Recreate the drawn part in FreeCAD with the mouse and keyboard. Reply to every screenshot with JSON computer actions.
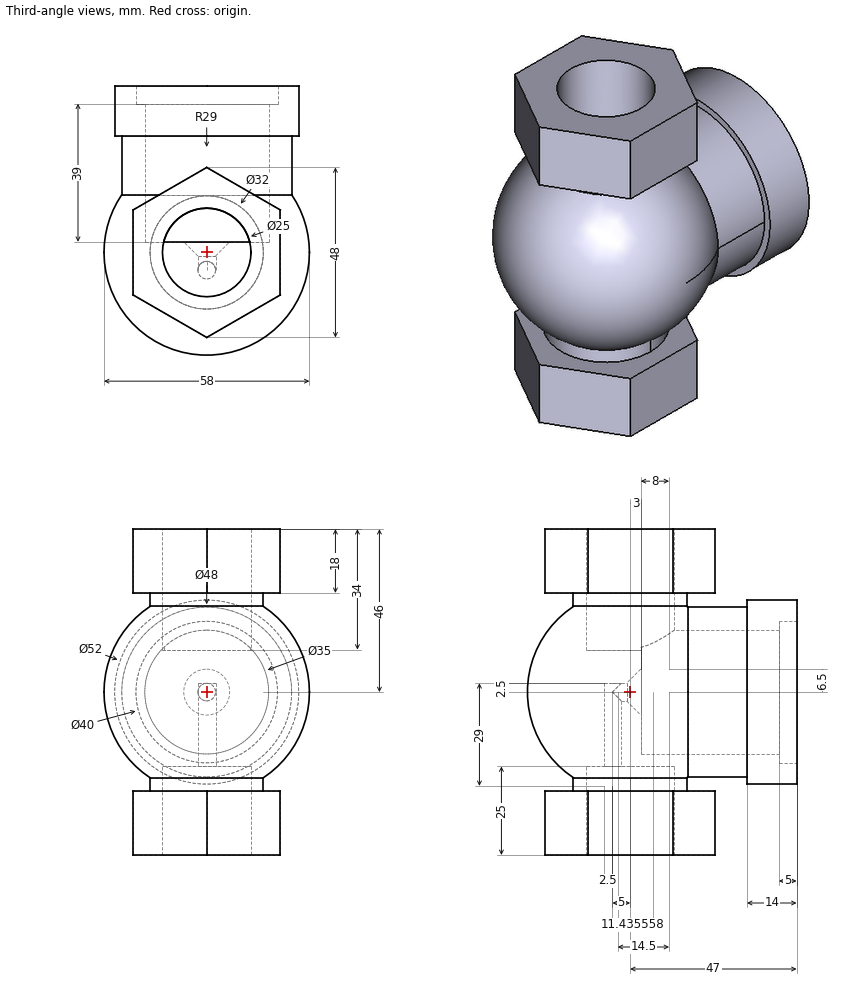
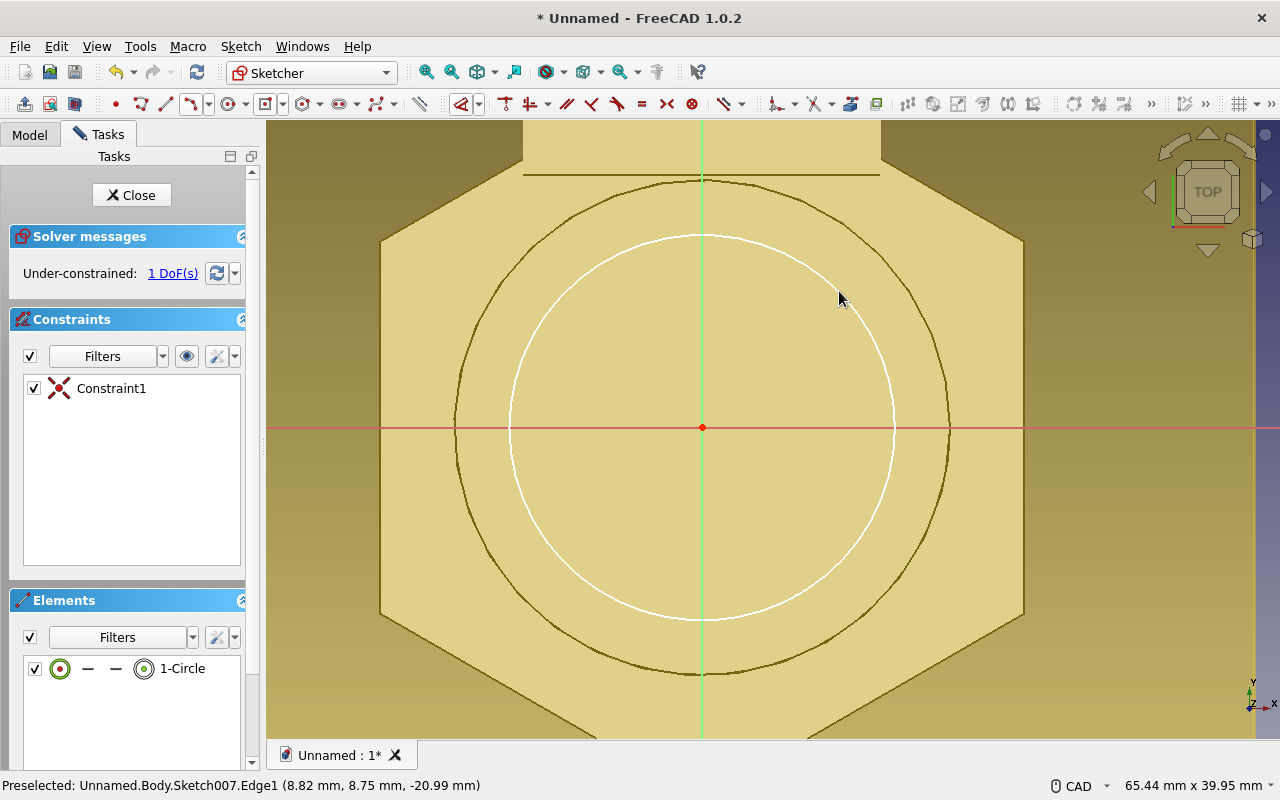
{"action": "left_click", "coordinate": [838, 291]}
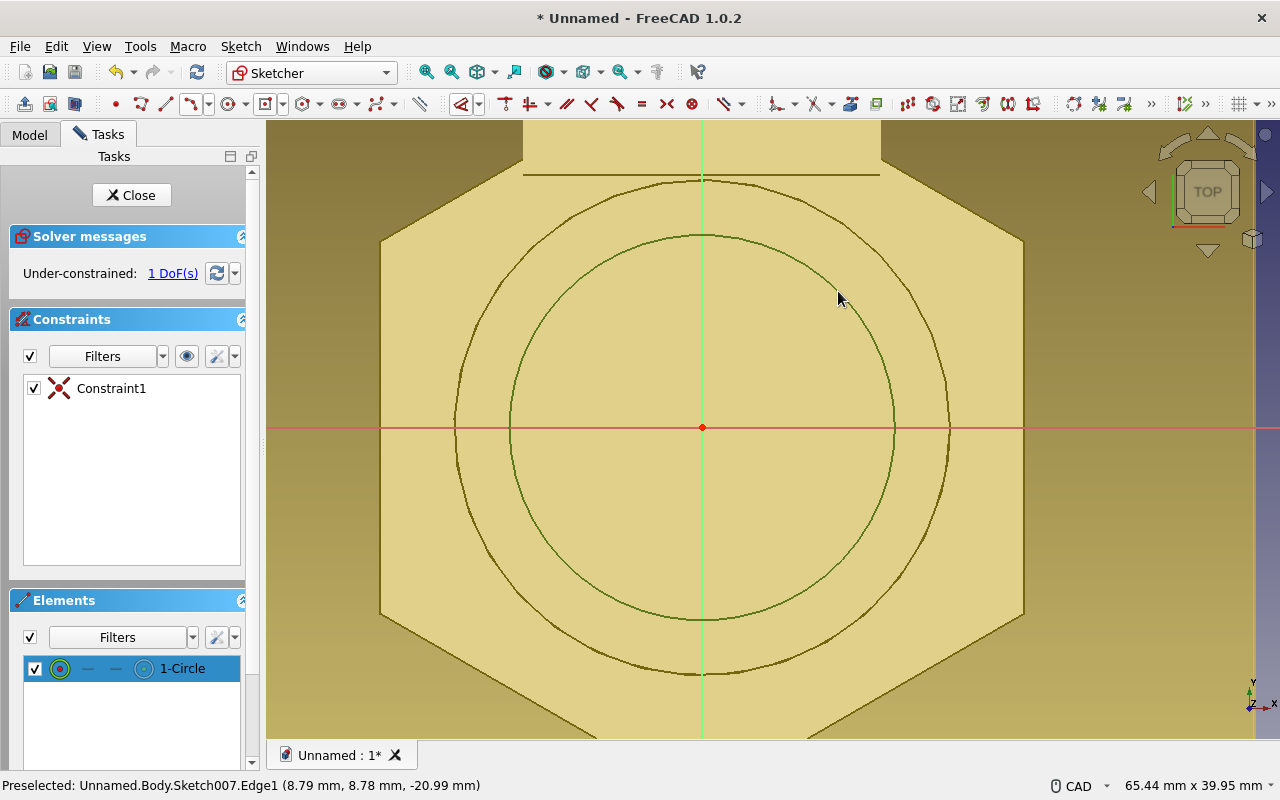
{"action": "key", "text": "k o"}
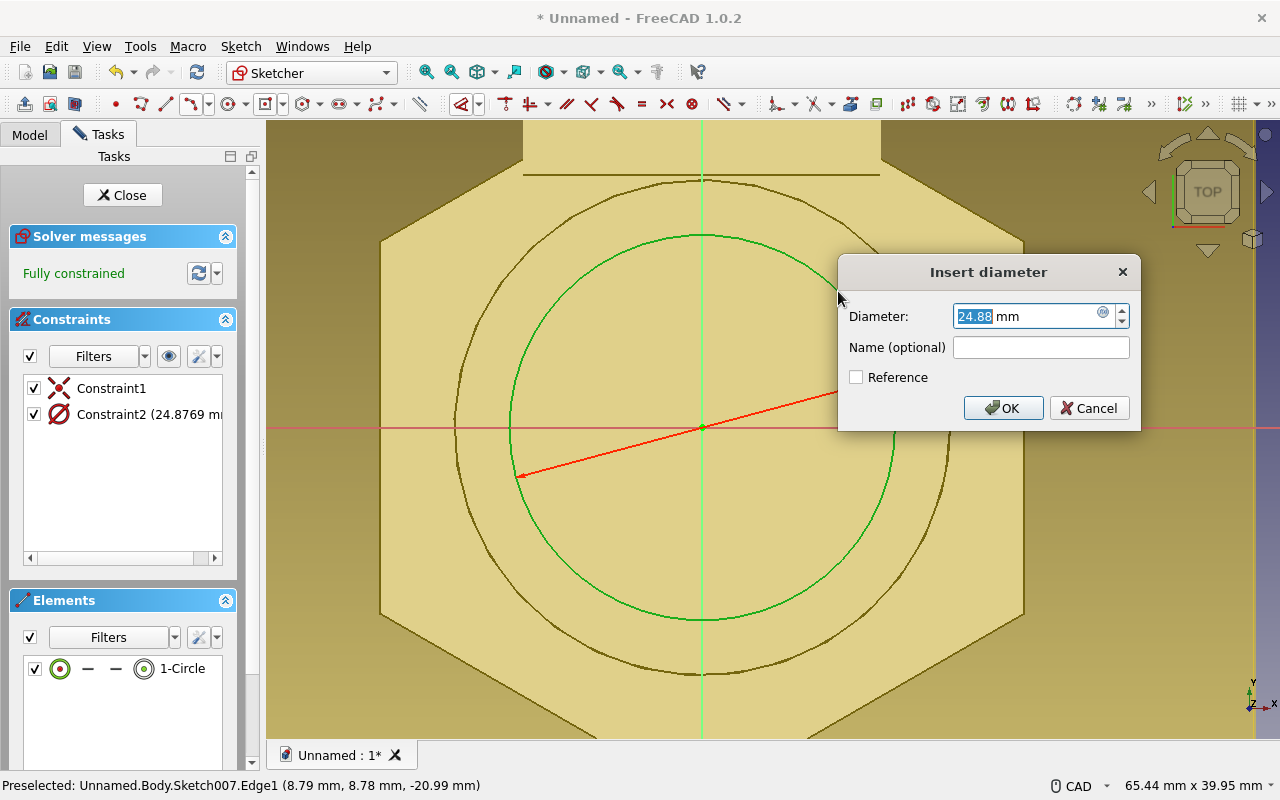
{"action": "type", "text": "25"}
{"action": "key", "text": "Return"}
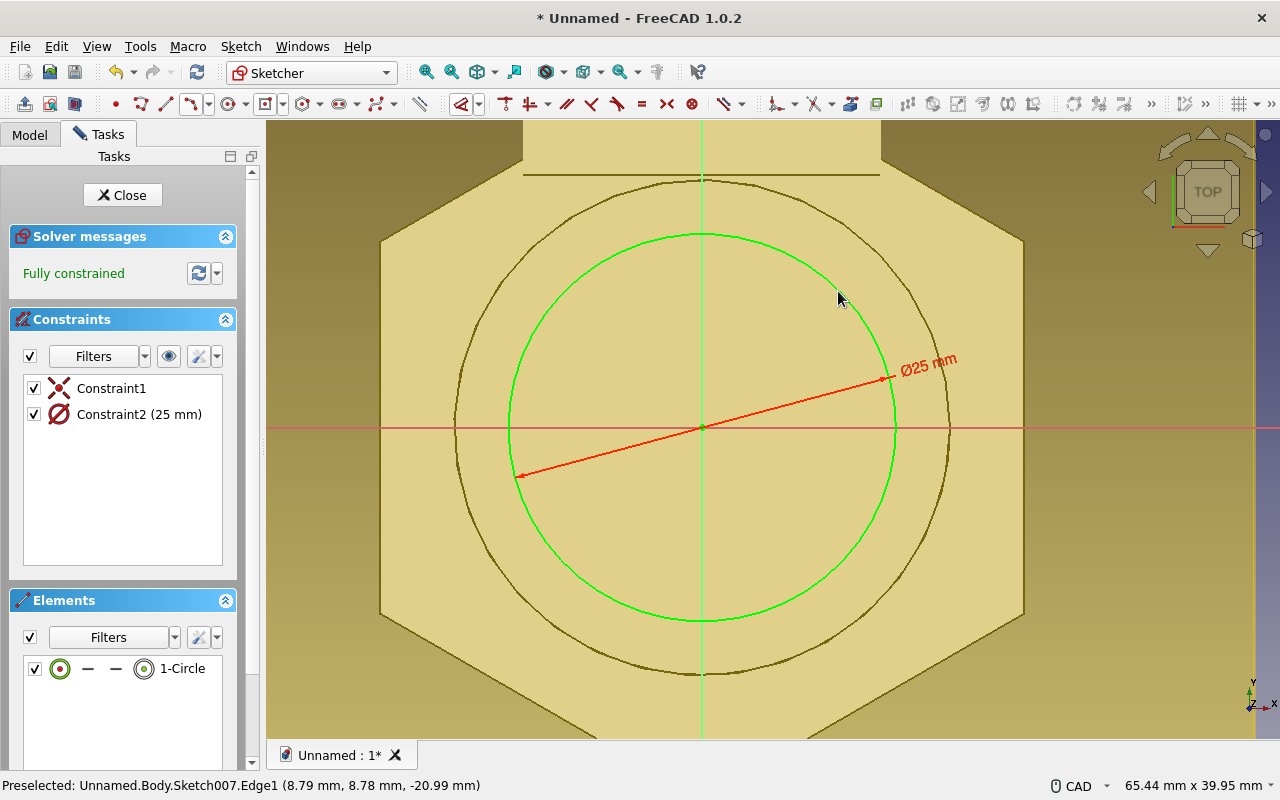
{"action": "left_click", "coordinate": [123, 195]}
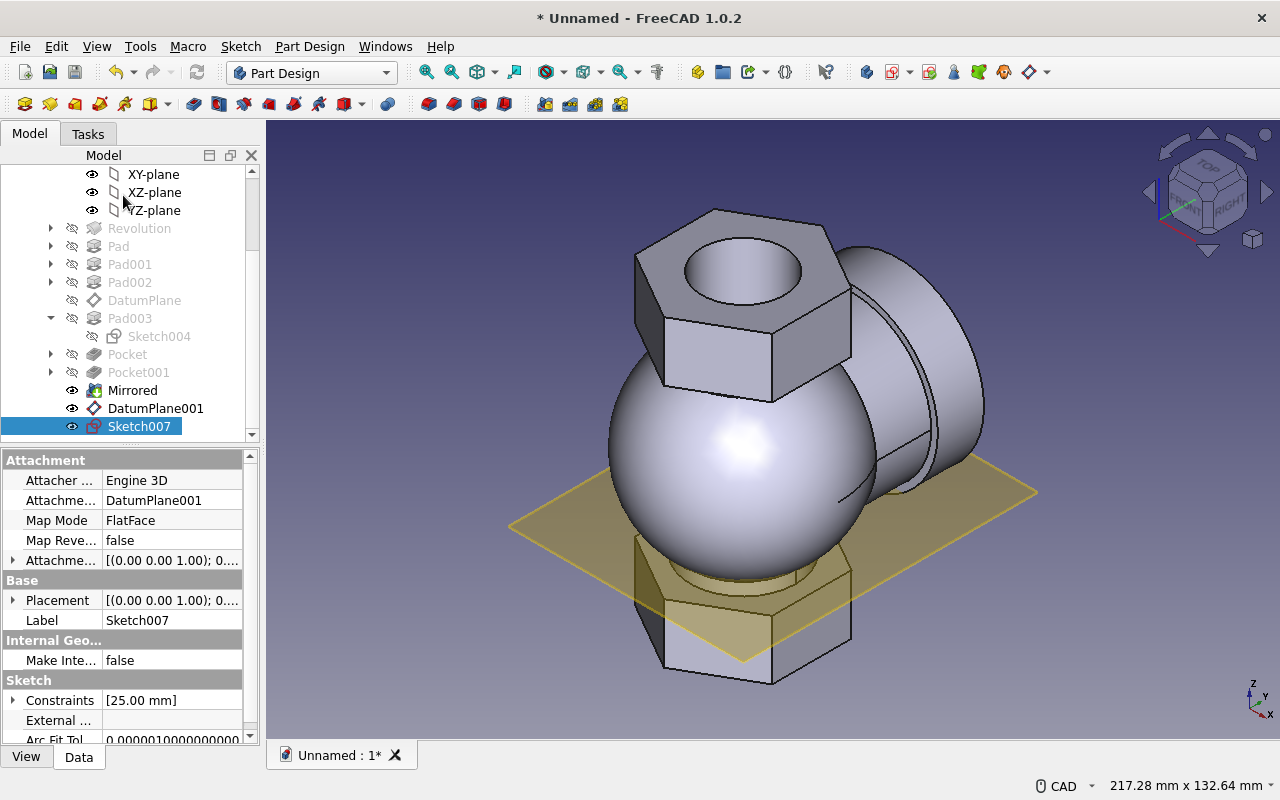
{"action": "left_click", "coordinate": [194, 104]}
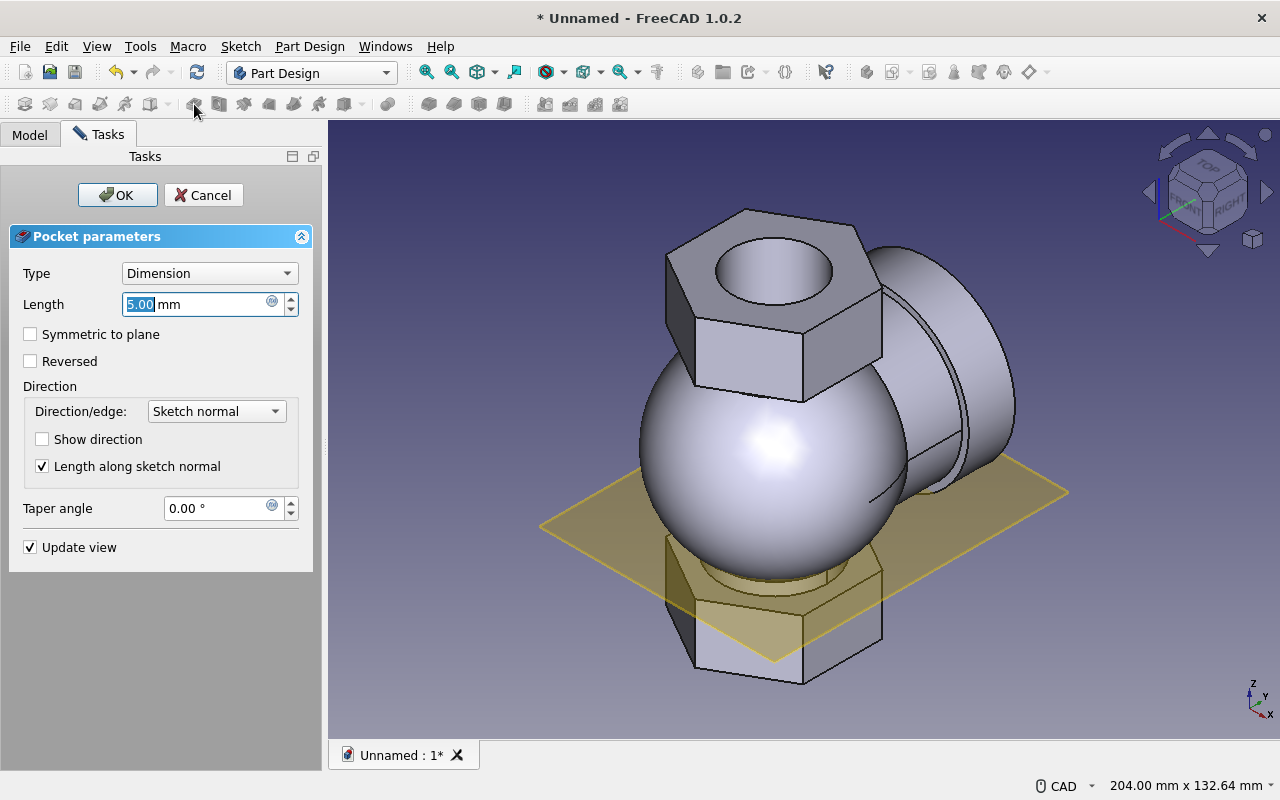
{"action": "type", "text": "25"}
{"action": "key", "text": "Tab"}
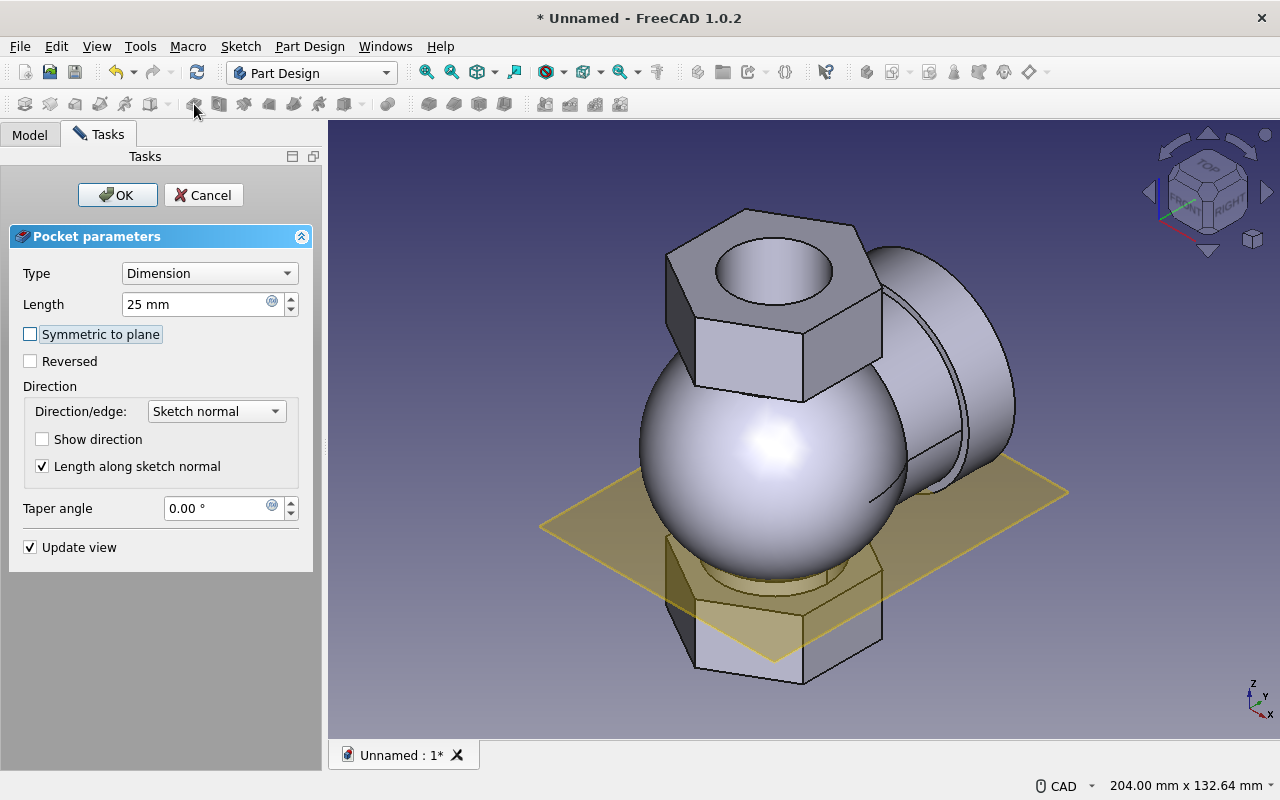
{"action": "left_click", "coordinate": [118, 195]}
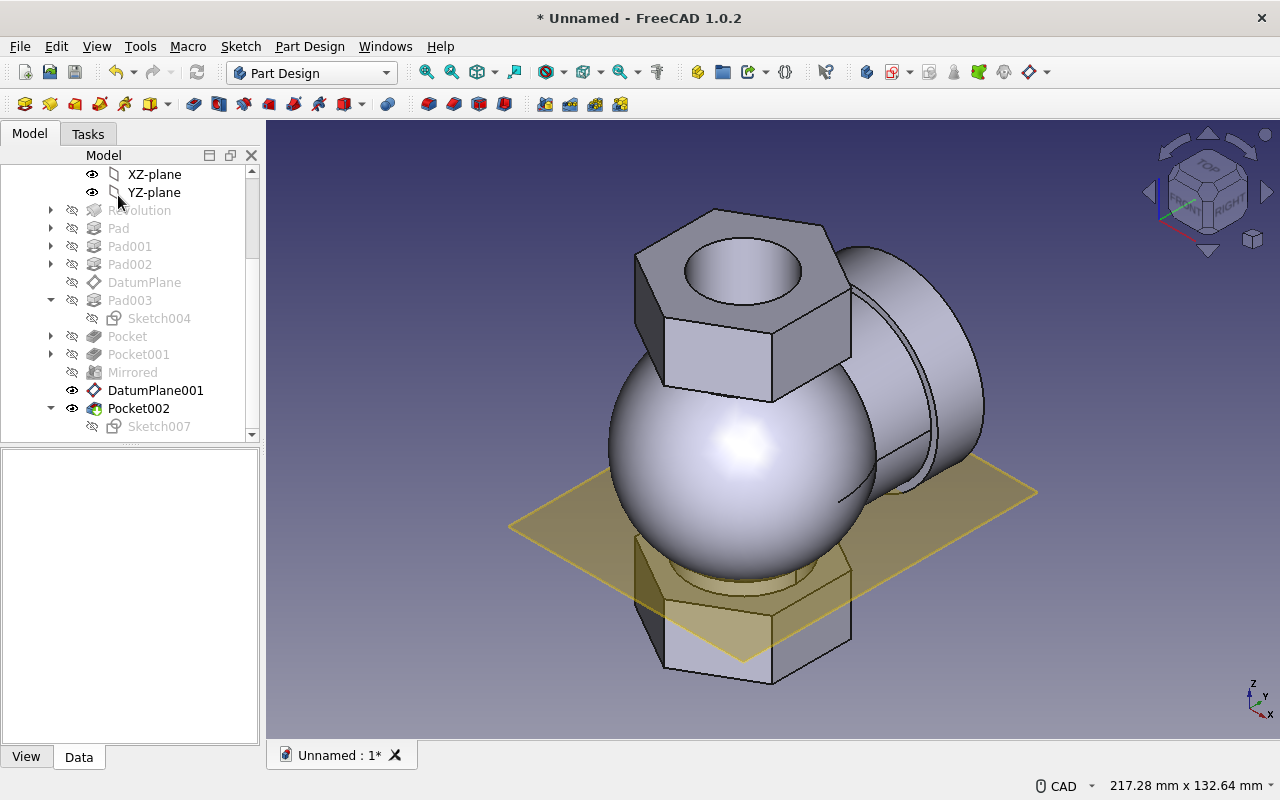
{"action": "left_click", "coordinate": [117, 390]}
{"action": "key", "text": "space"}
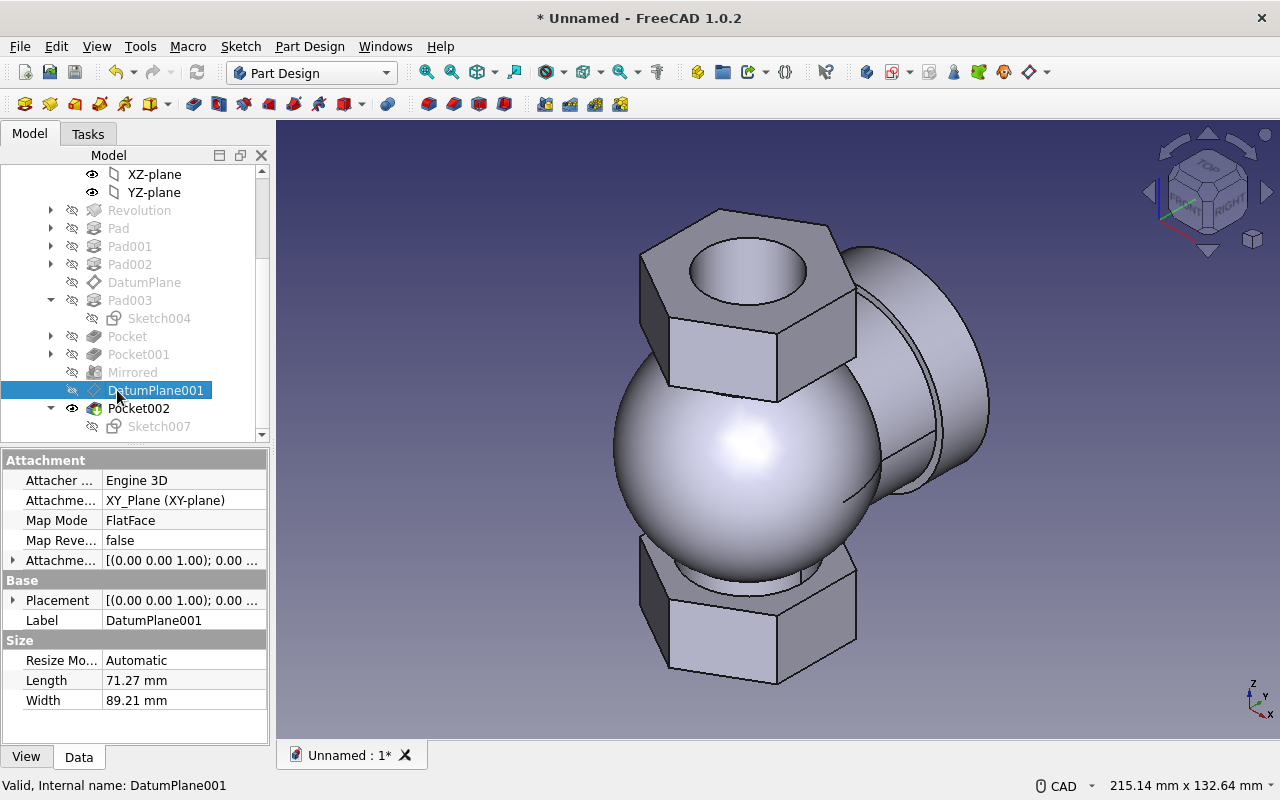
{"action": "key", "text": "4"}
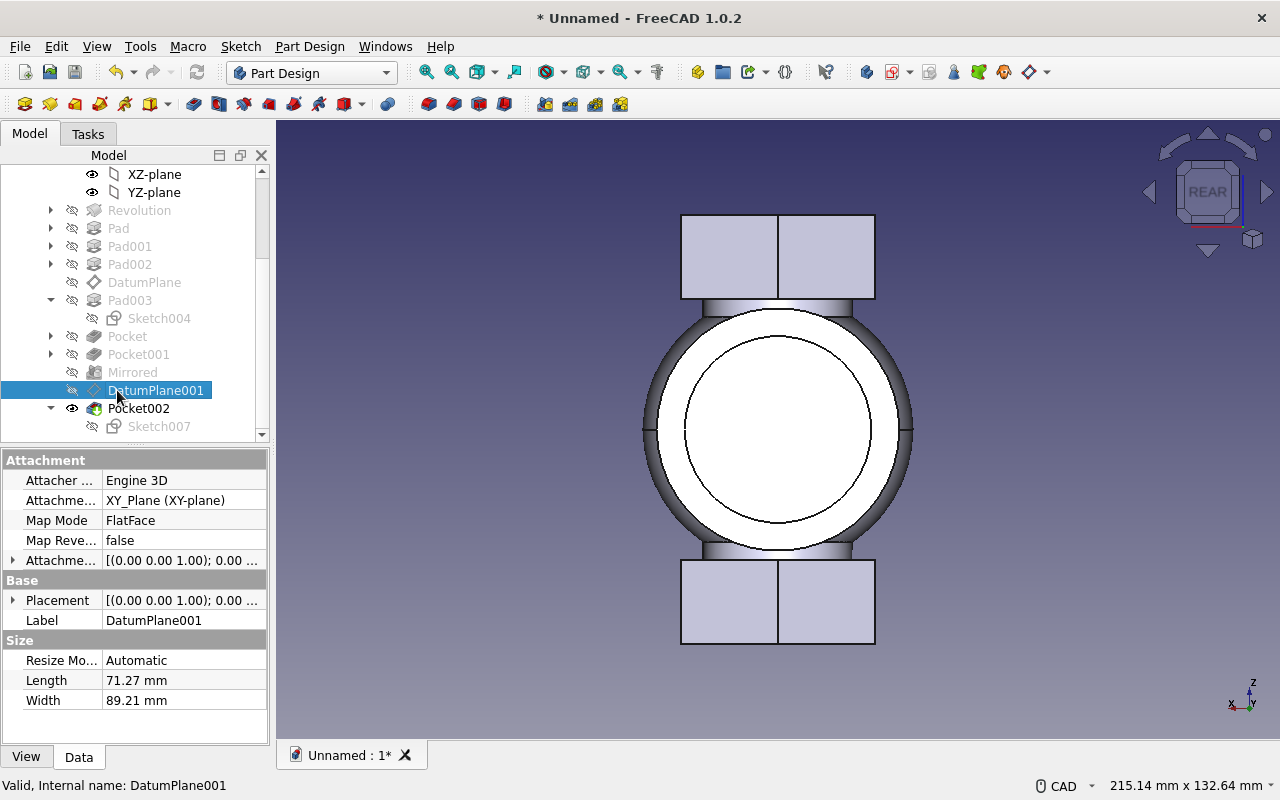
{"action": "left_click", "coordinate": [778, 428]}